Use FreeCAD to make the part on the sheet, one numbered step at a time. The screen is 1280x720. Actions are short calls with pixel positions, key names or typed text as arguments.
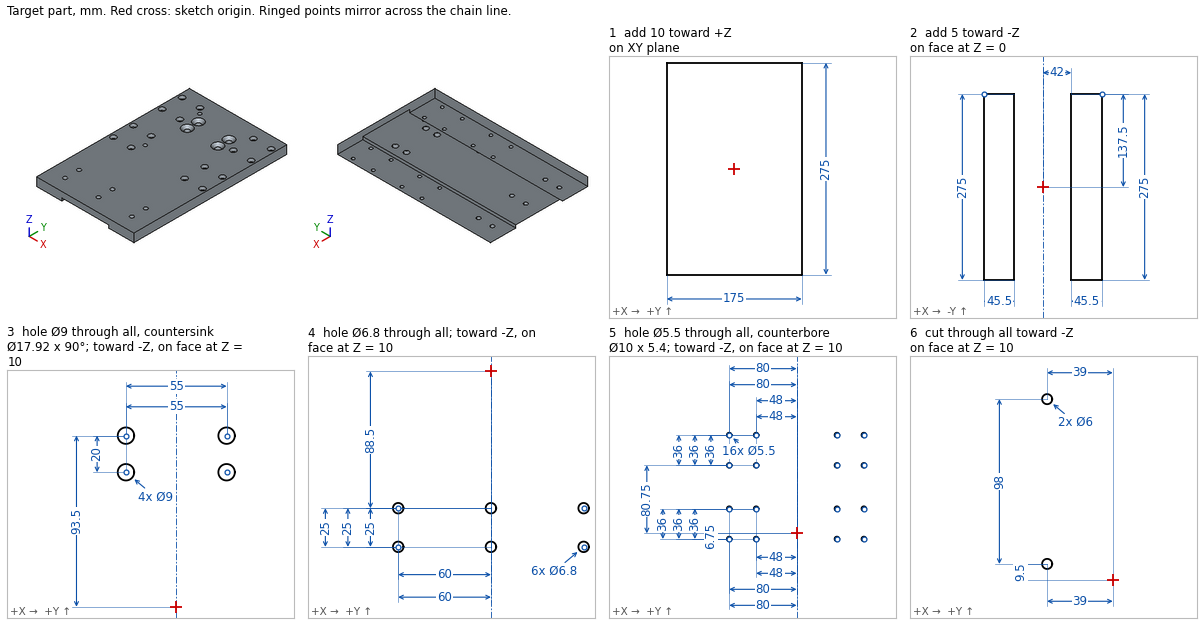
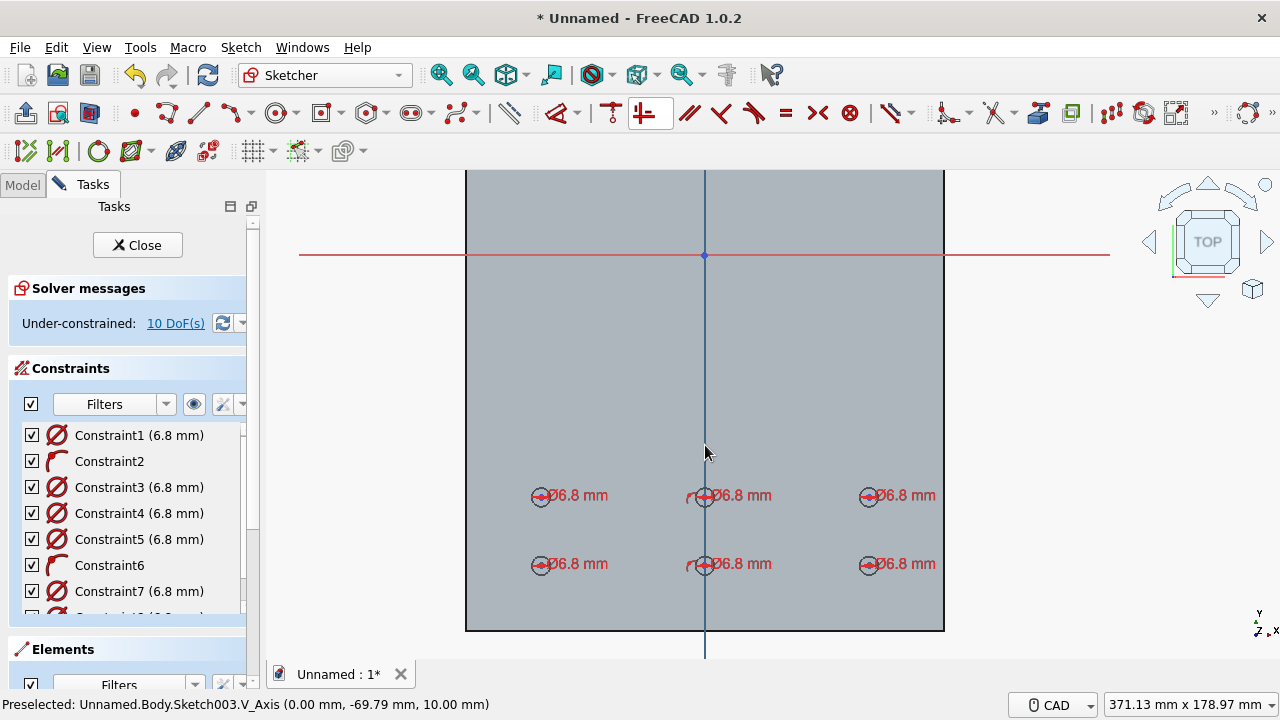
key(s)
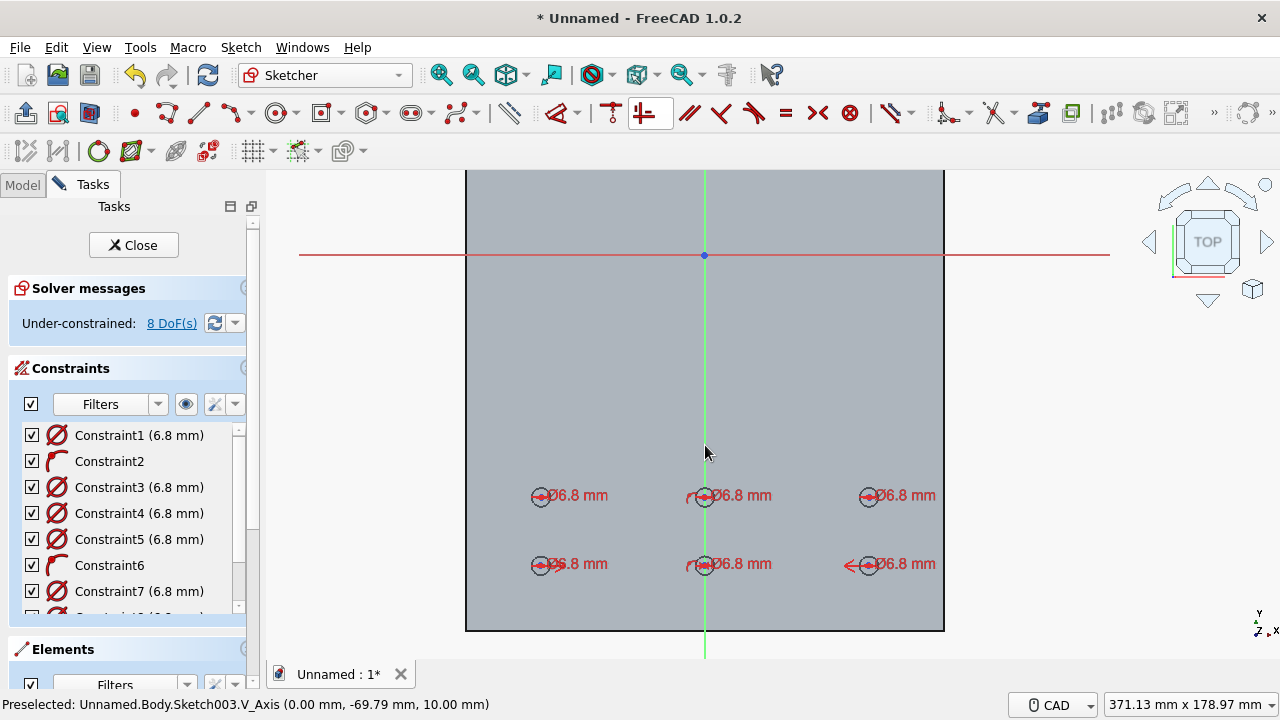
click(541, 497)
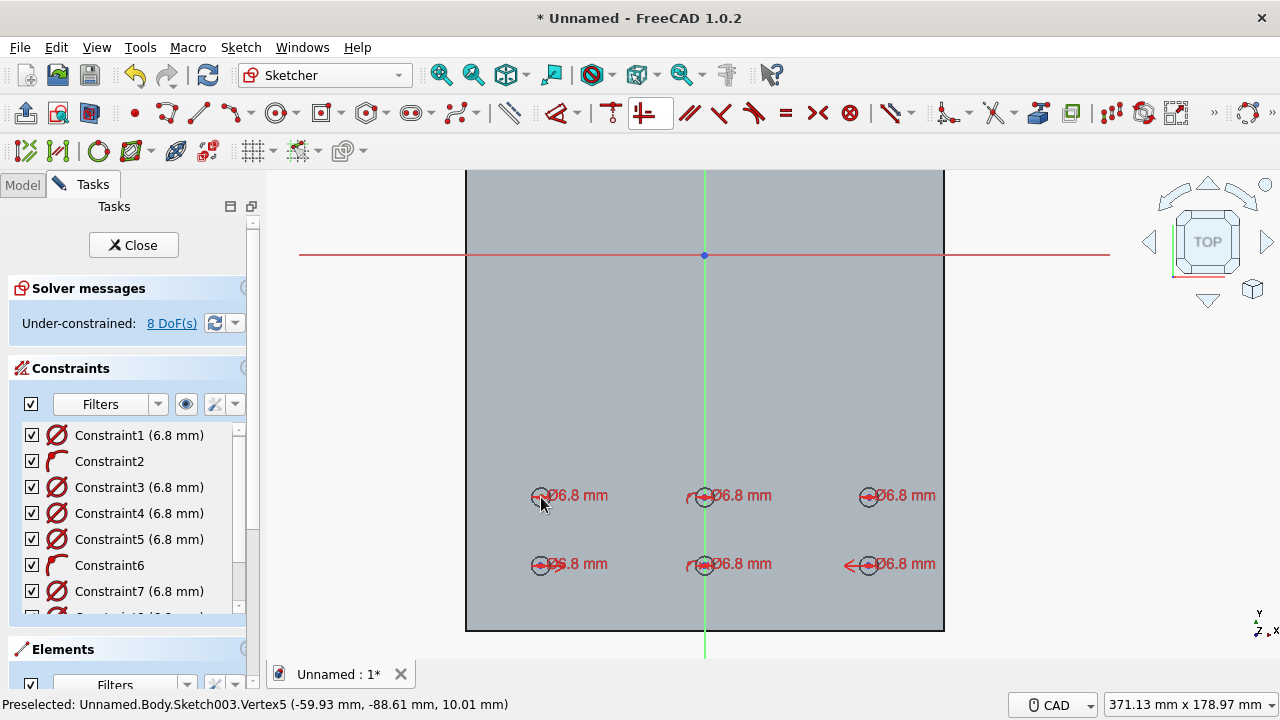
click(869, 497)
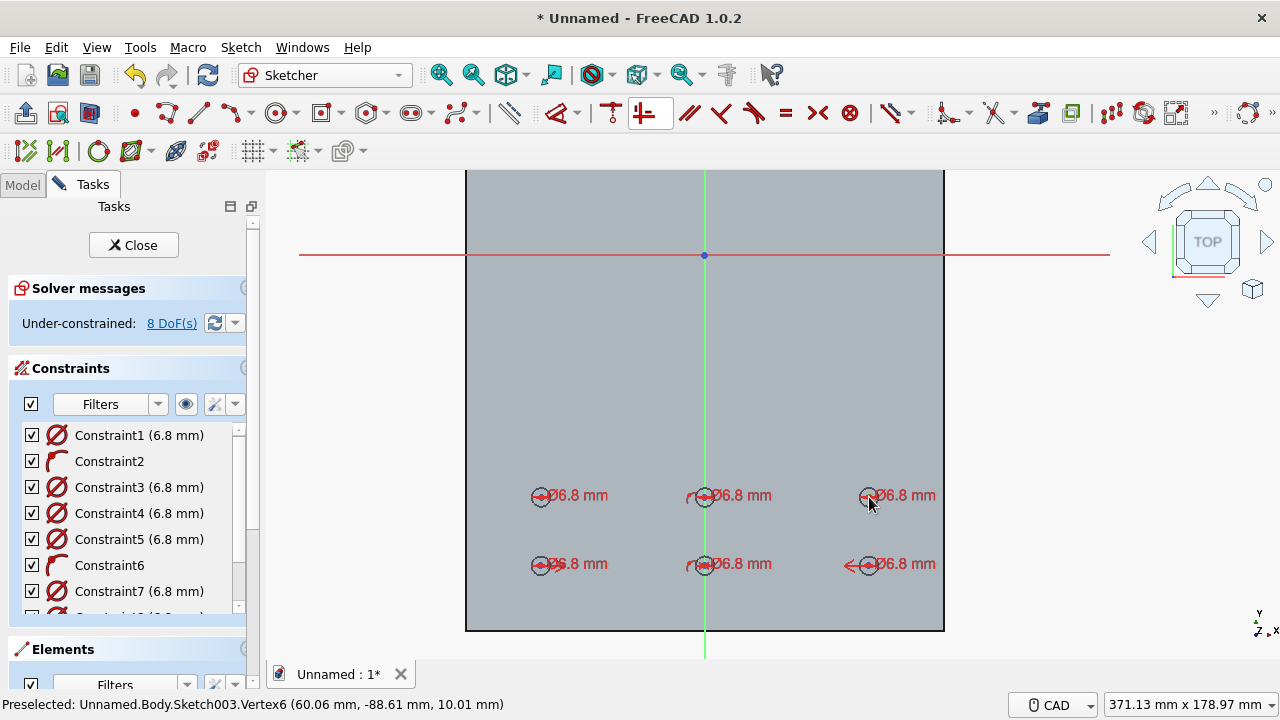
click(705, 445)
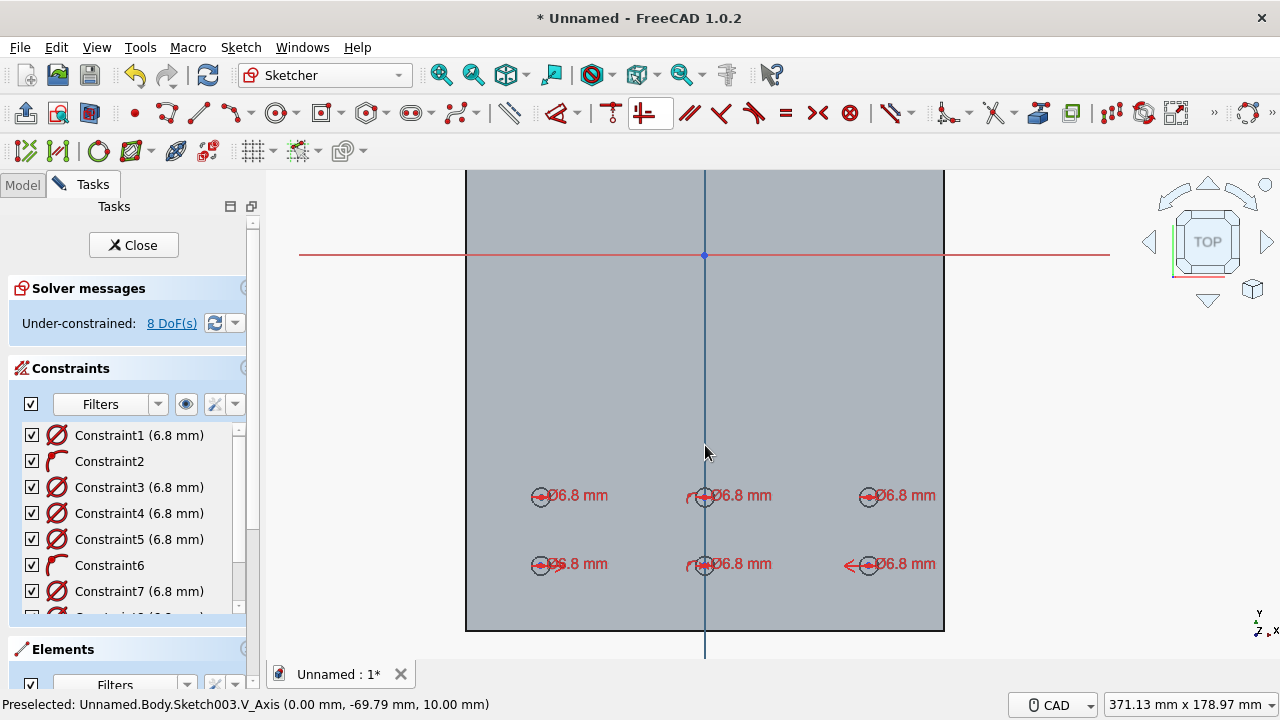
key(s)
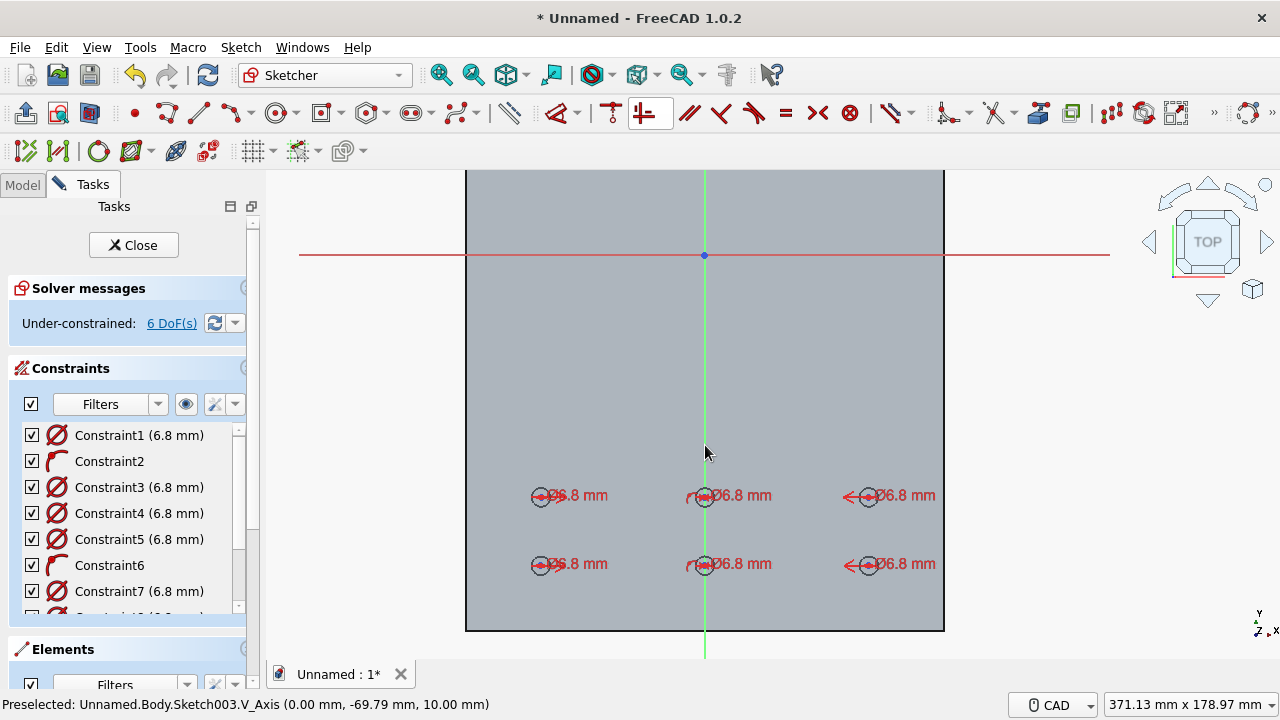
key(d)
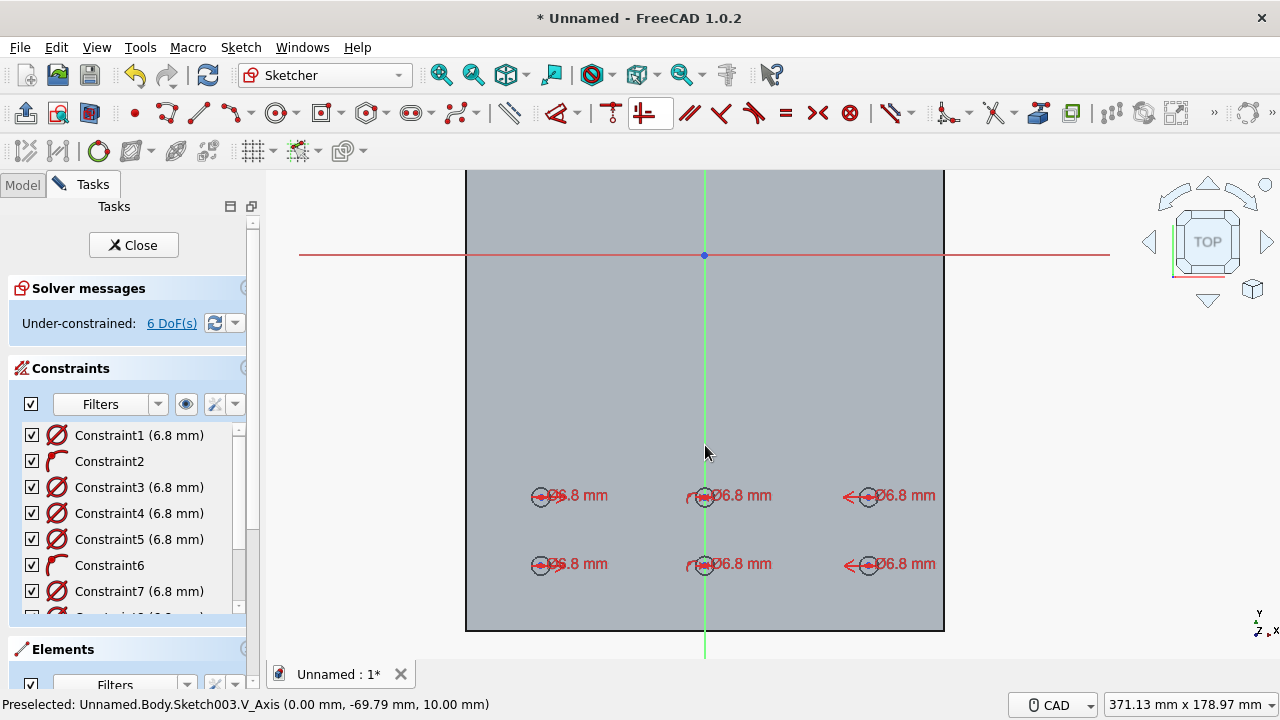
click(541, 566)
click(623, 221)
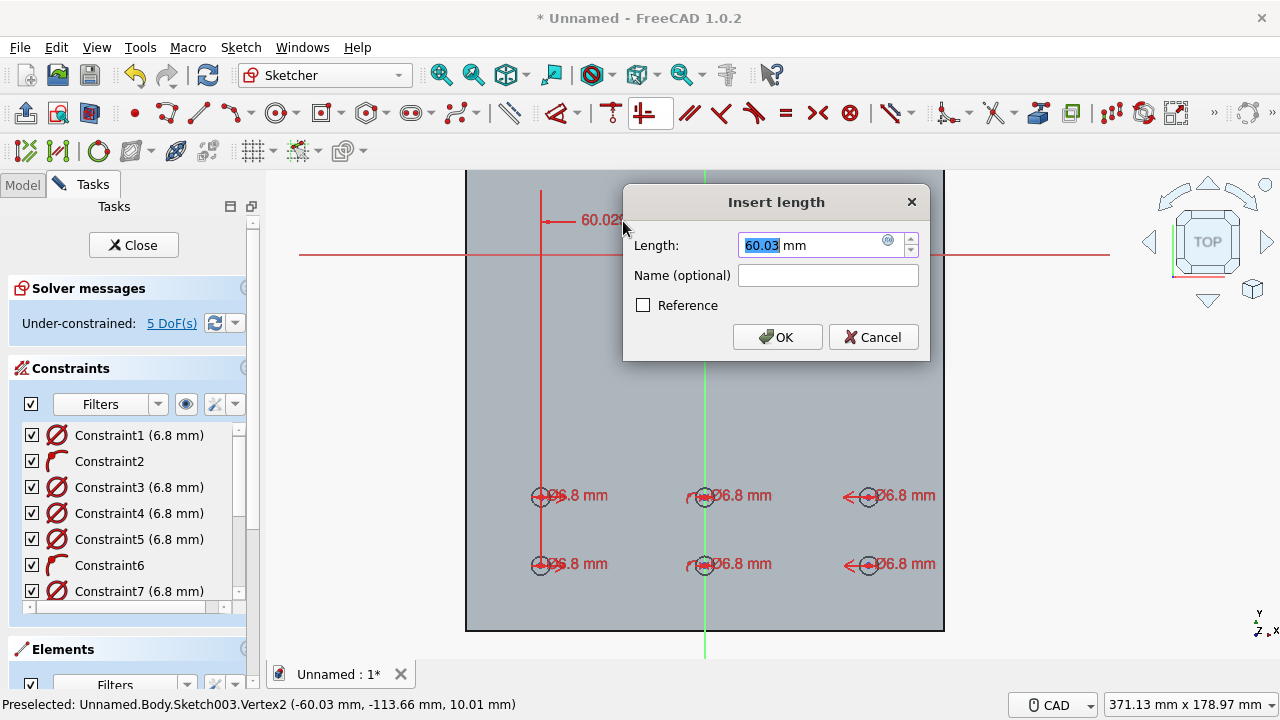
text(60)
key(Return)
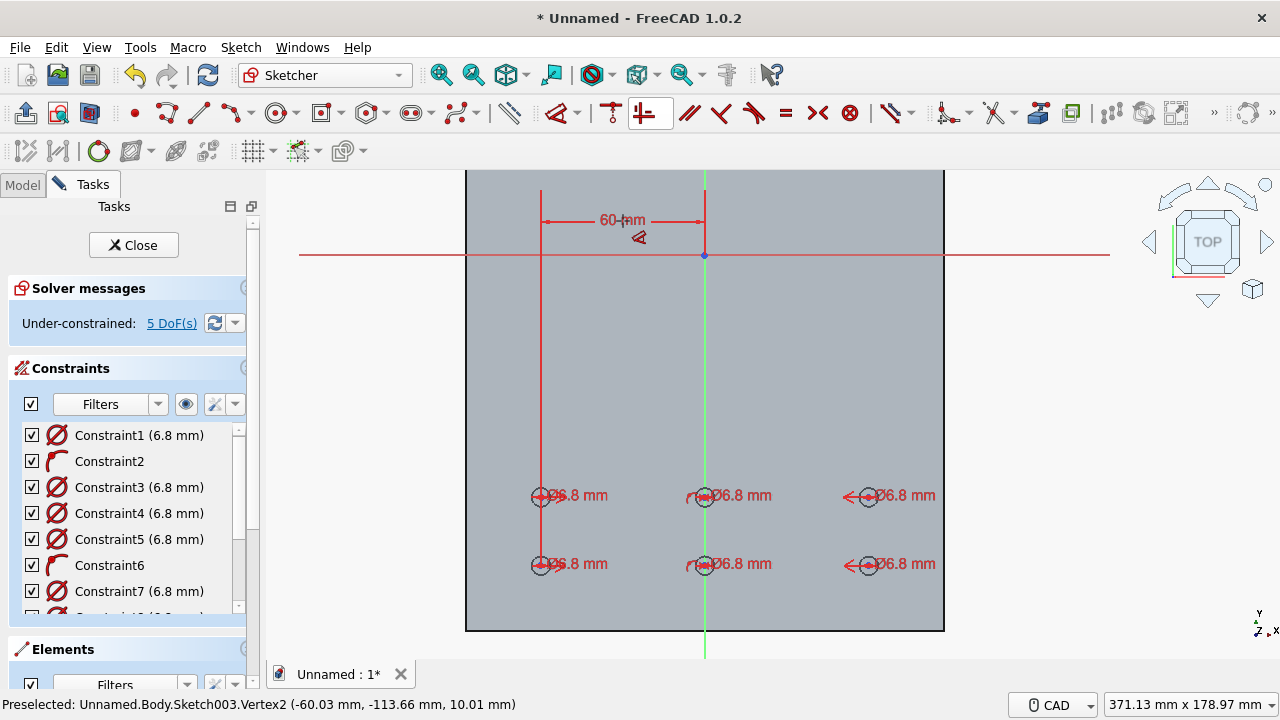
click(541, 497)
click(623, 531)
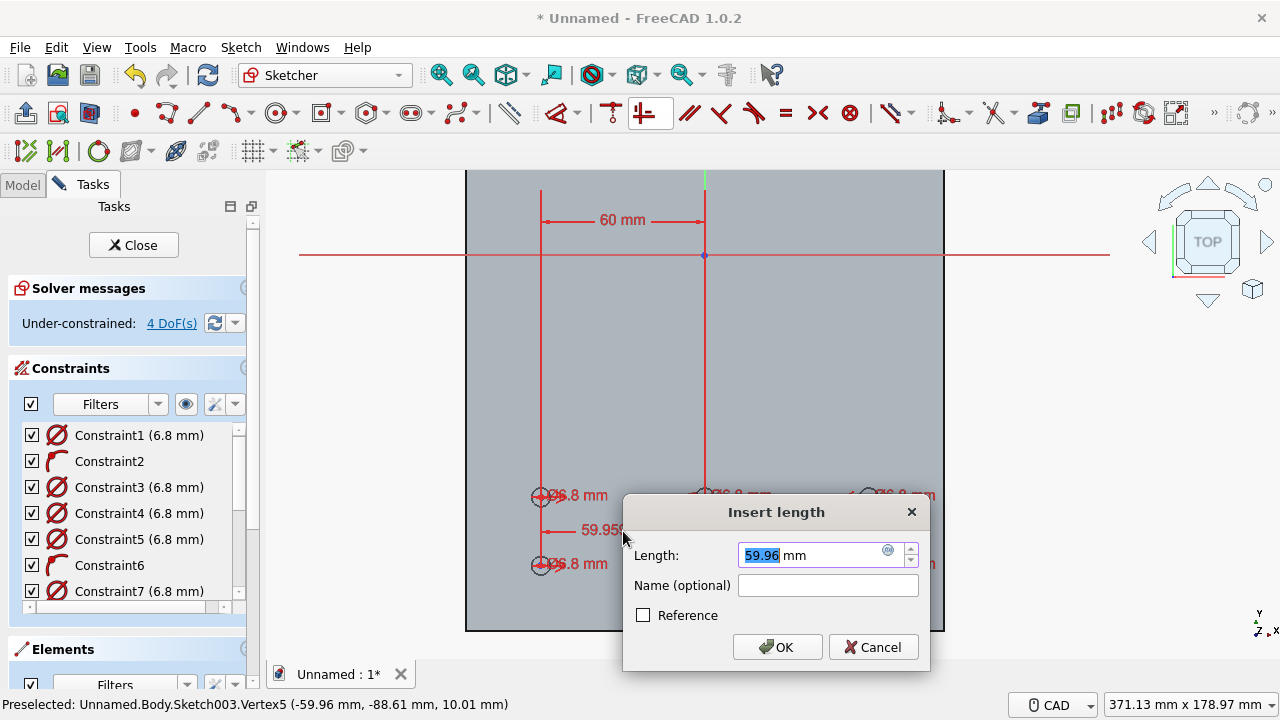
text(60)
key(Return)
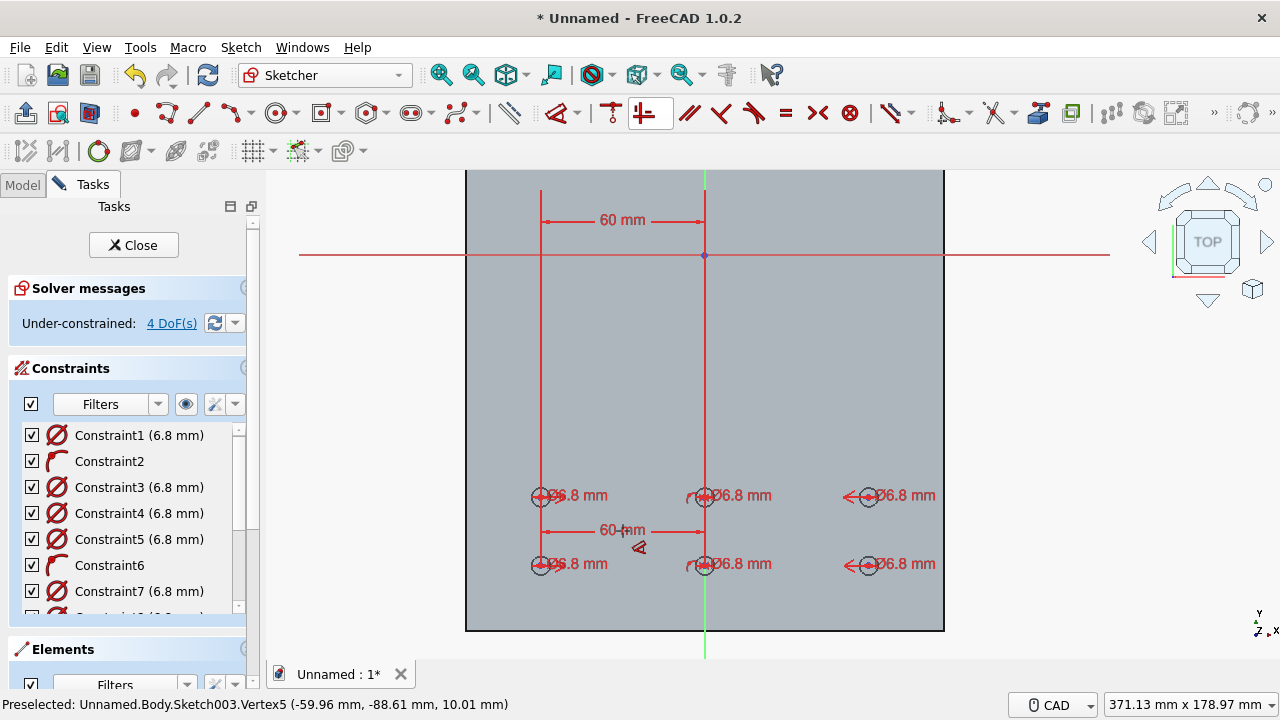
click(705, 566)